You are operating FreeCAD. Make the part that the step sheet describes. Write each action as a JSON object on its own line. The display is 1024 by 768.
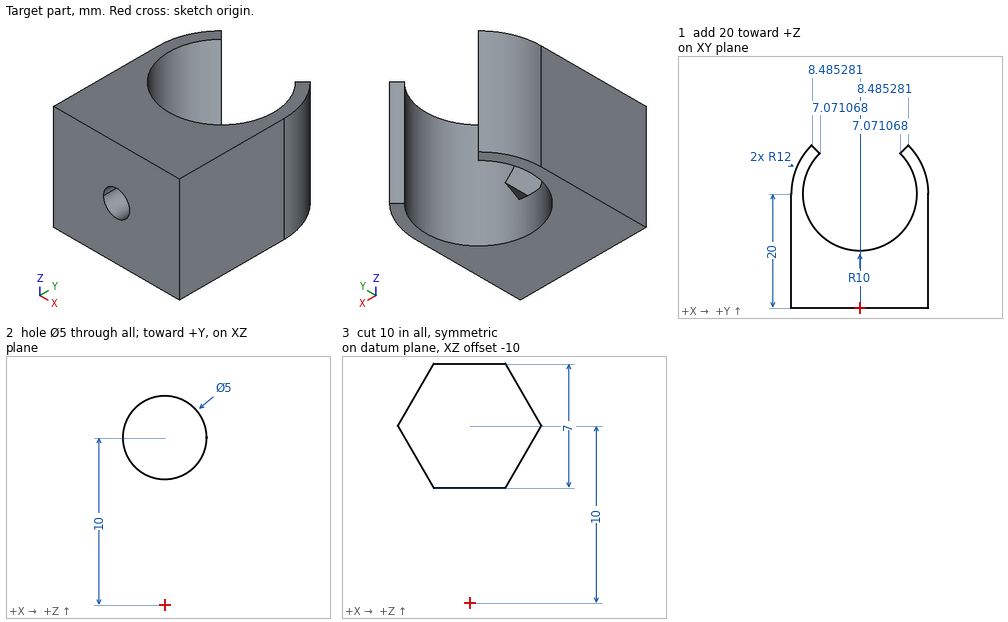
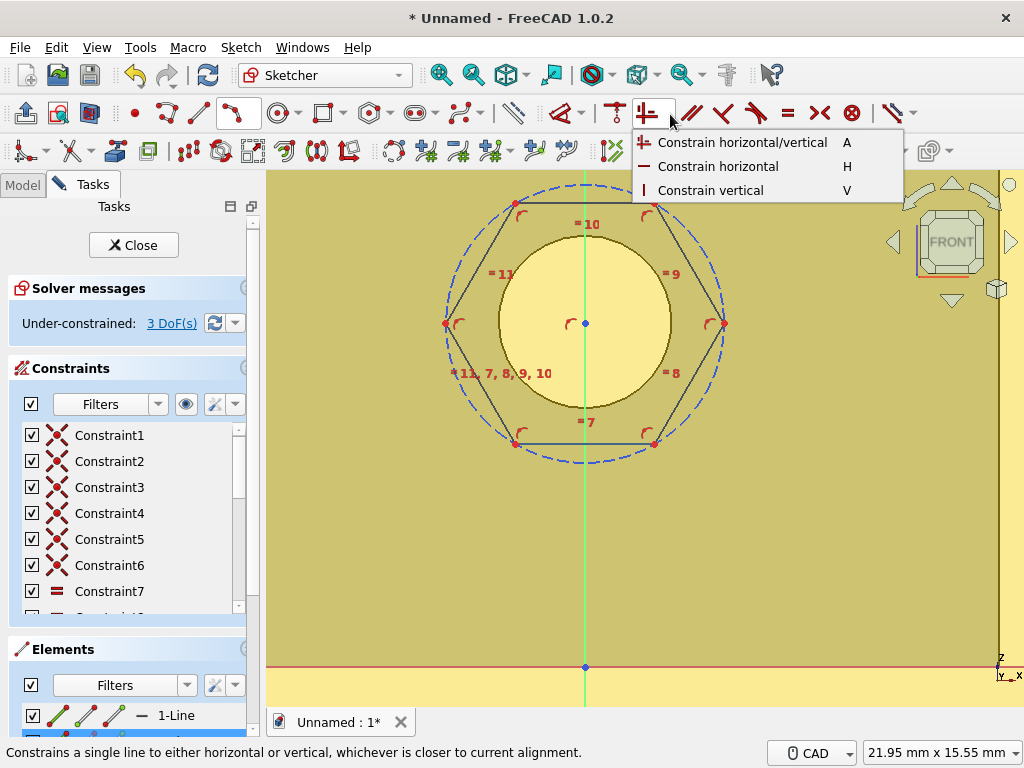
{"action": "left_click", "coordinate": [768, 166]}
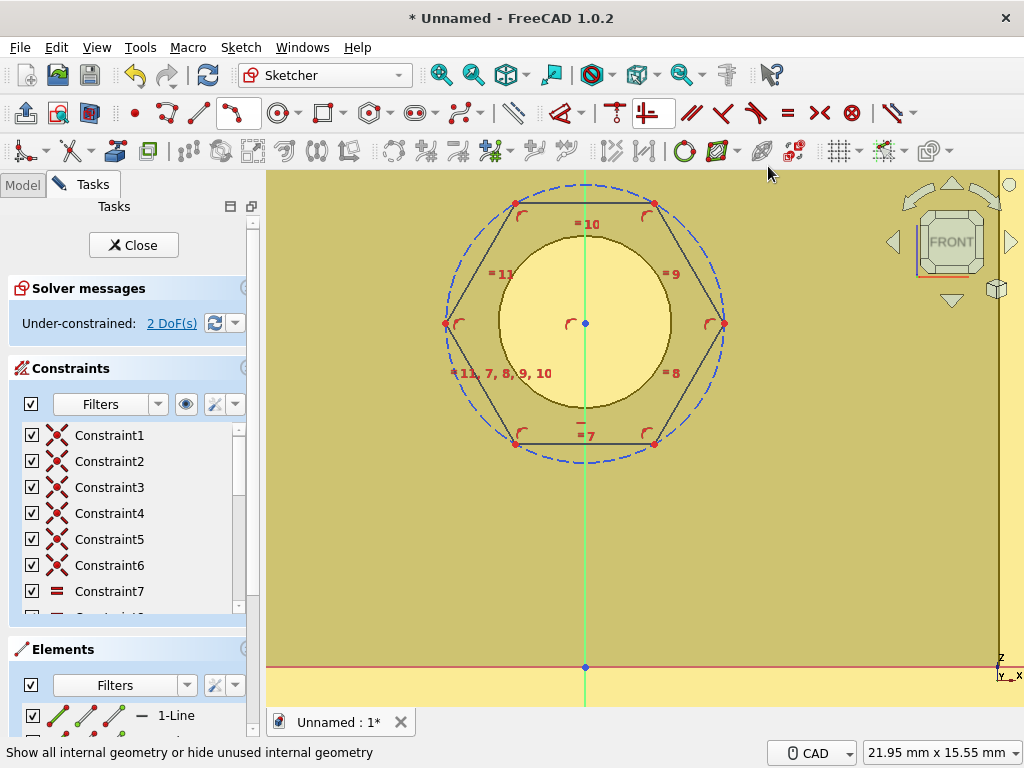
{"action": "left_click", "coordinate": [560, 114]}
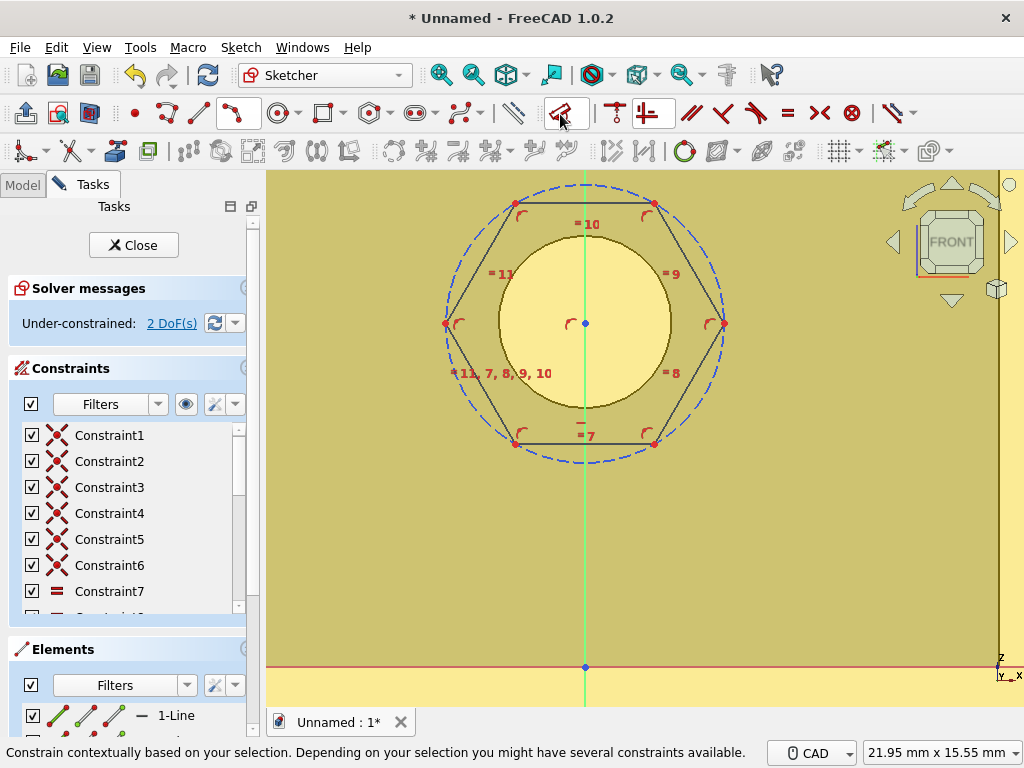
{"action": "left_click", "coordinate": [515, 444]}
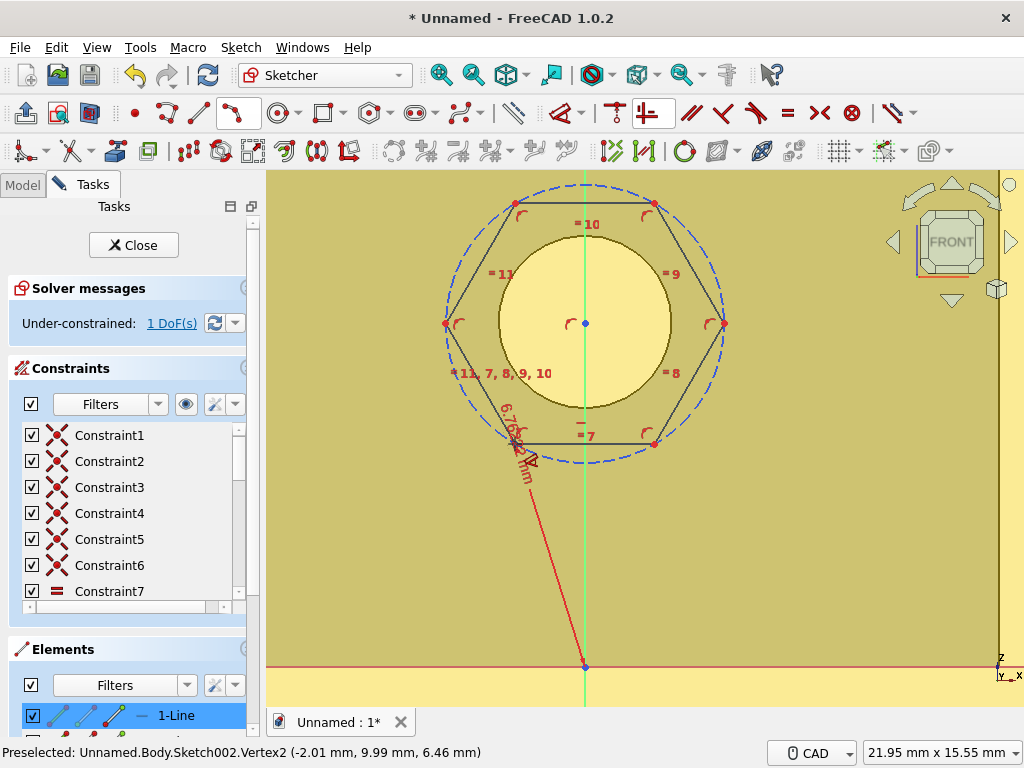
{"action": "left_click", "coordinate": [655, 203]}
{"action": "left_click", "coordinate": [689, 324]}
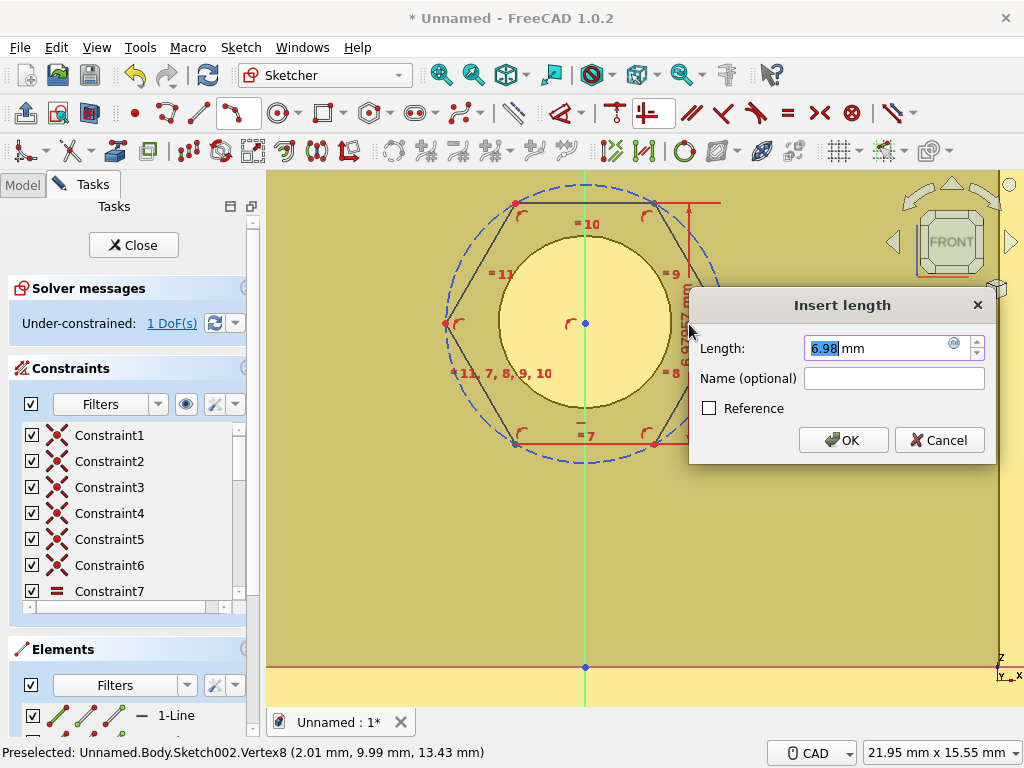
{"action": "type", "text": "7"}
{"action": "key", "text": "Return"}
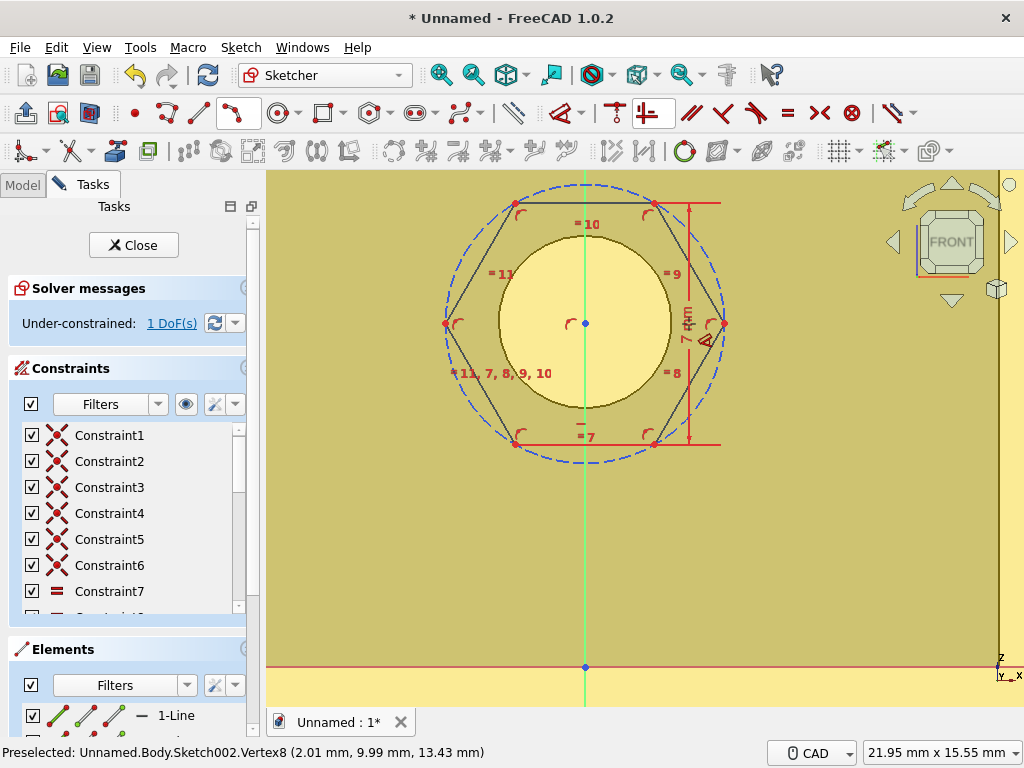
{"action": "left_click", "coordinate": [585, 324]}
{"action": "left_click", "coordinate": [619, 496]}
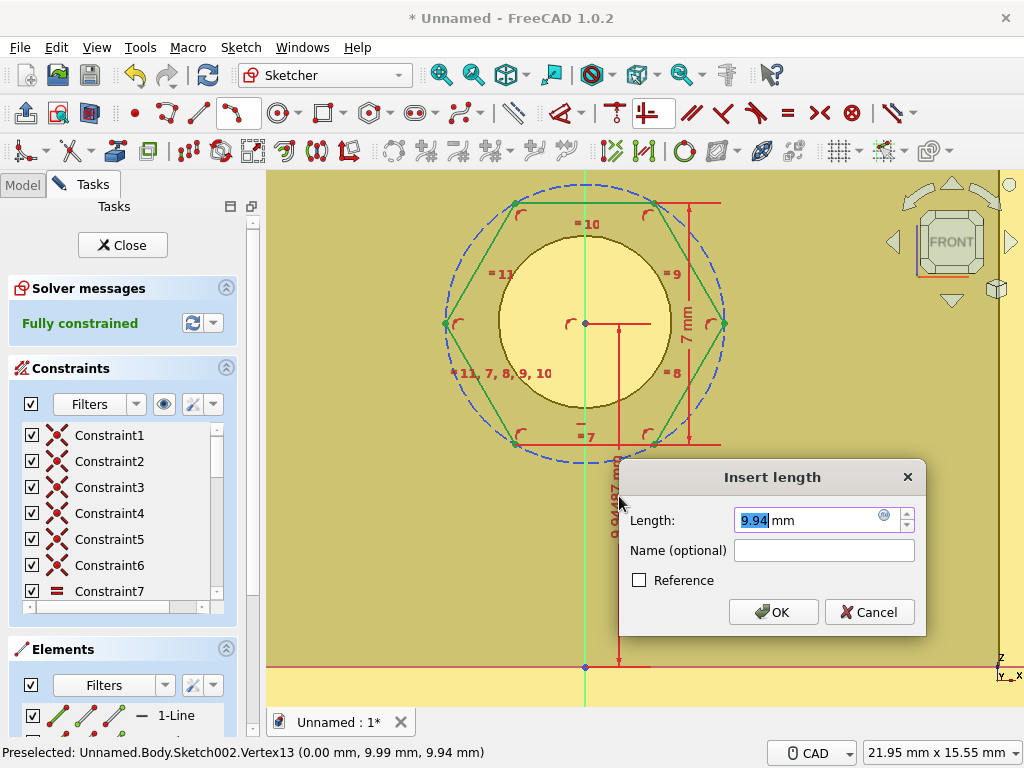
{"action": "type", "text": "10"}
{"action": "key", "text": "Return"}
{"action": "key", "text": "Escape"}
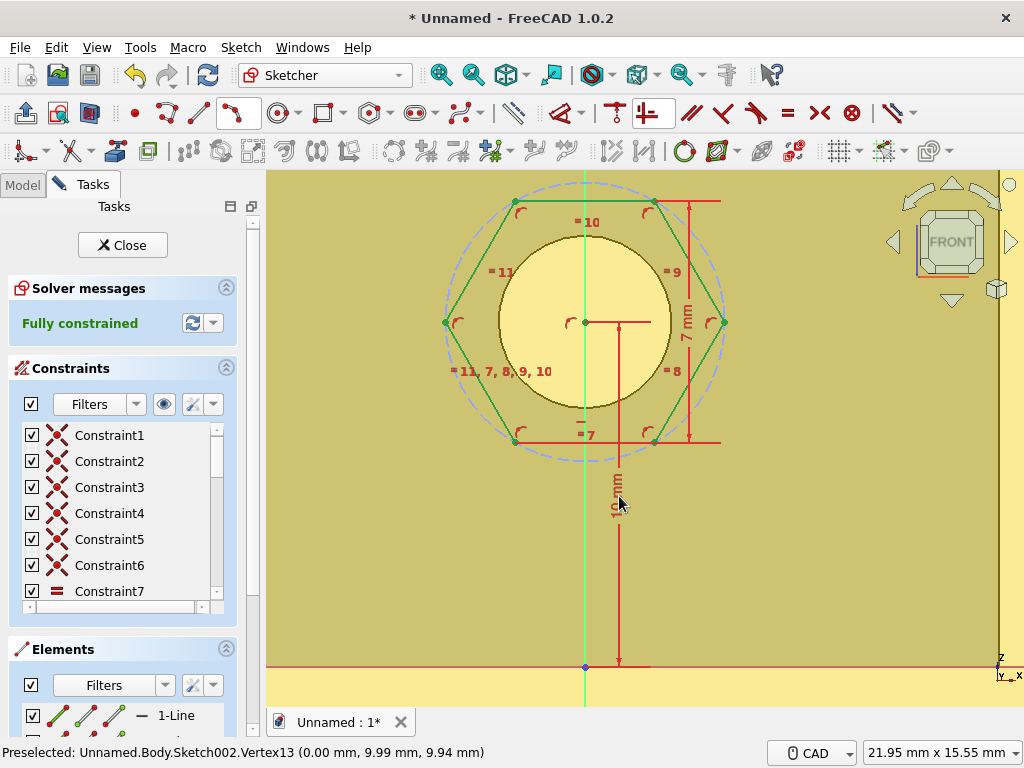
{"action": "left_click", "coordinate": [123, 245]}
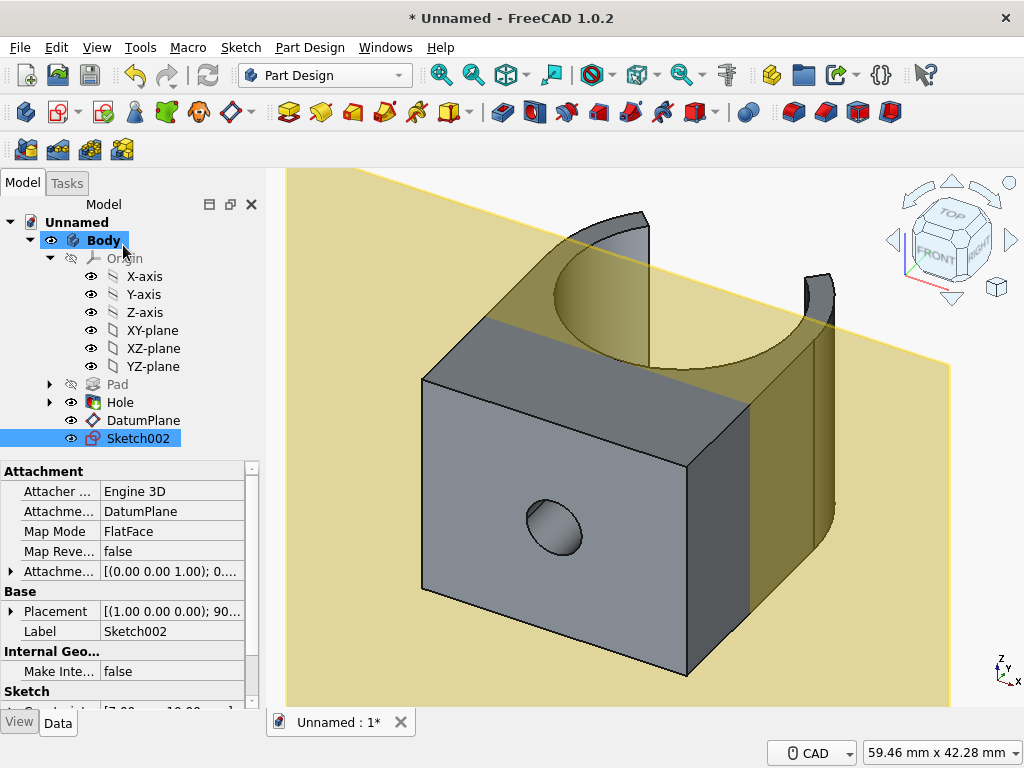
{"action": "left_click", "coordinate": [504, 112]}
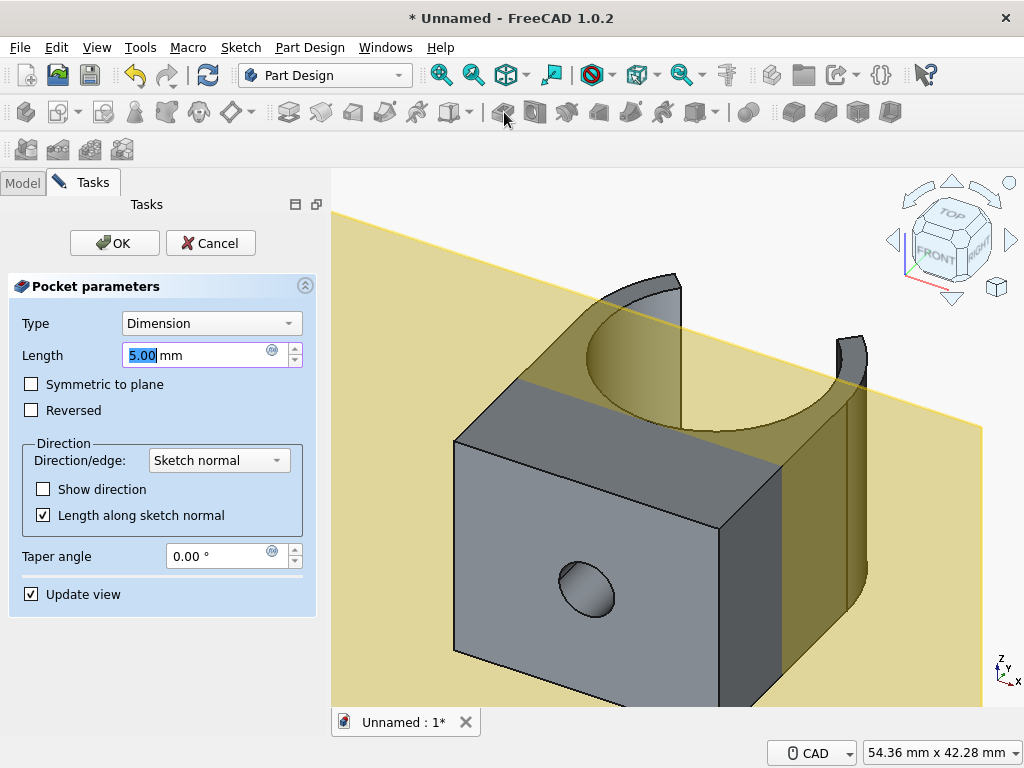
{"action": "type", "text": "10"}
{"action": "key", "text": "Tab"}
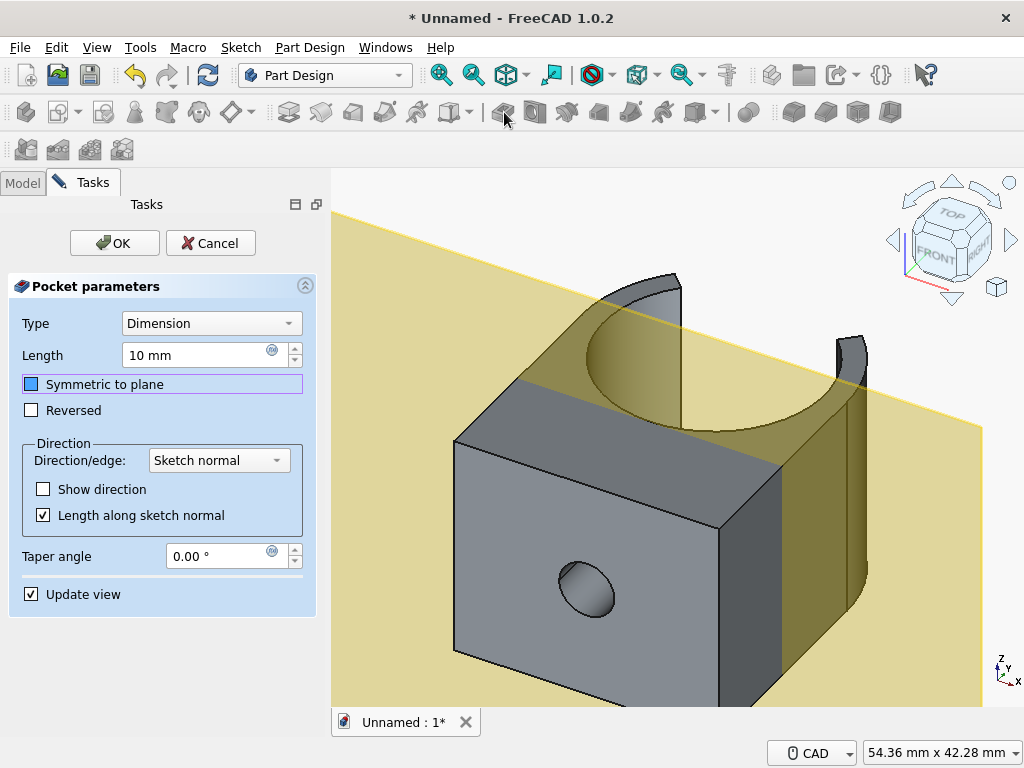
{"action": "left_click", "coordinate": [30, 384]}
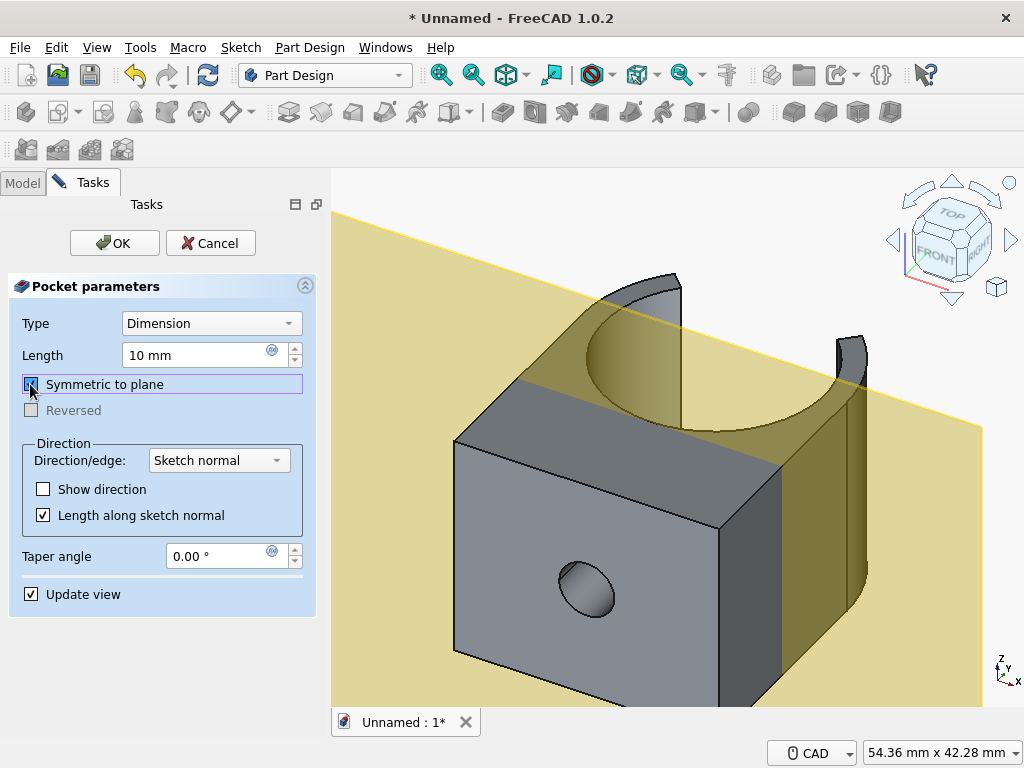
{"action": "left_click", "coordinate": [115, 243]}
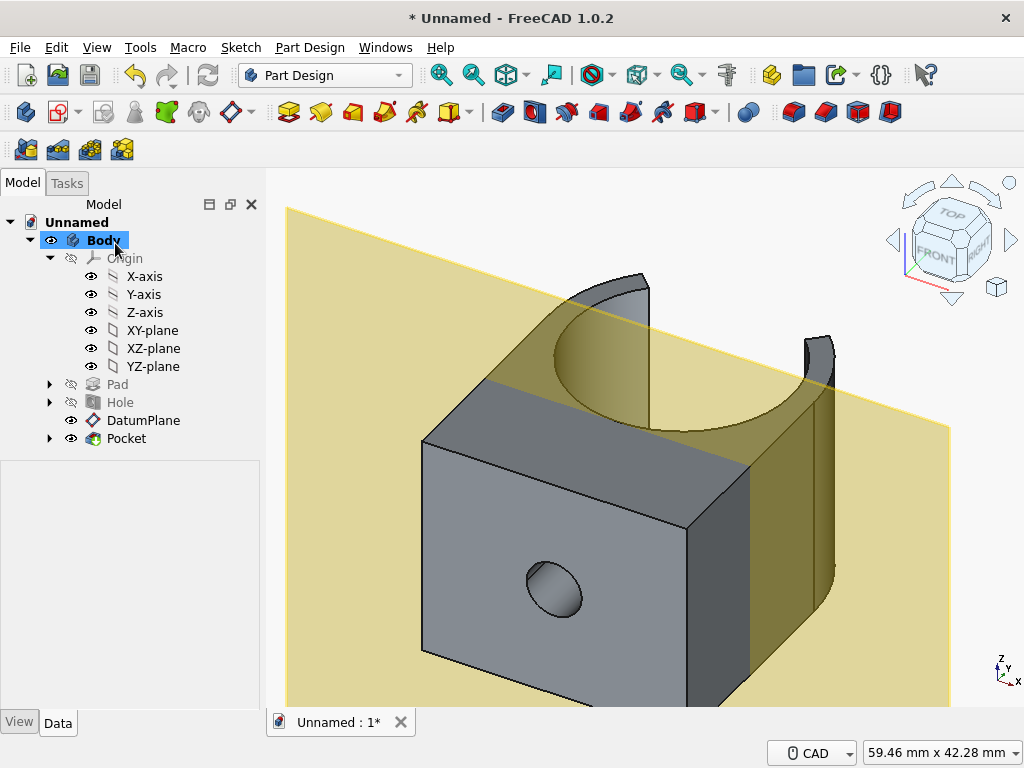
{"action": "left_click", "coordinate": [116, 420]}
{"action": "key", "text": "space"}